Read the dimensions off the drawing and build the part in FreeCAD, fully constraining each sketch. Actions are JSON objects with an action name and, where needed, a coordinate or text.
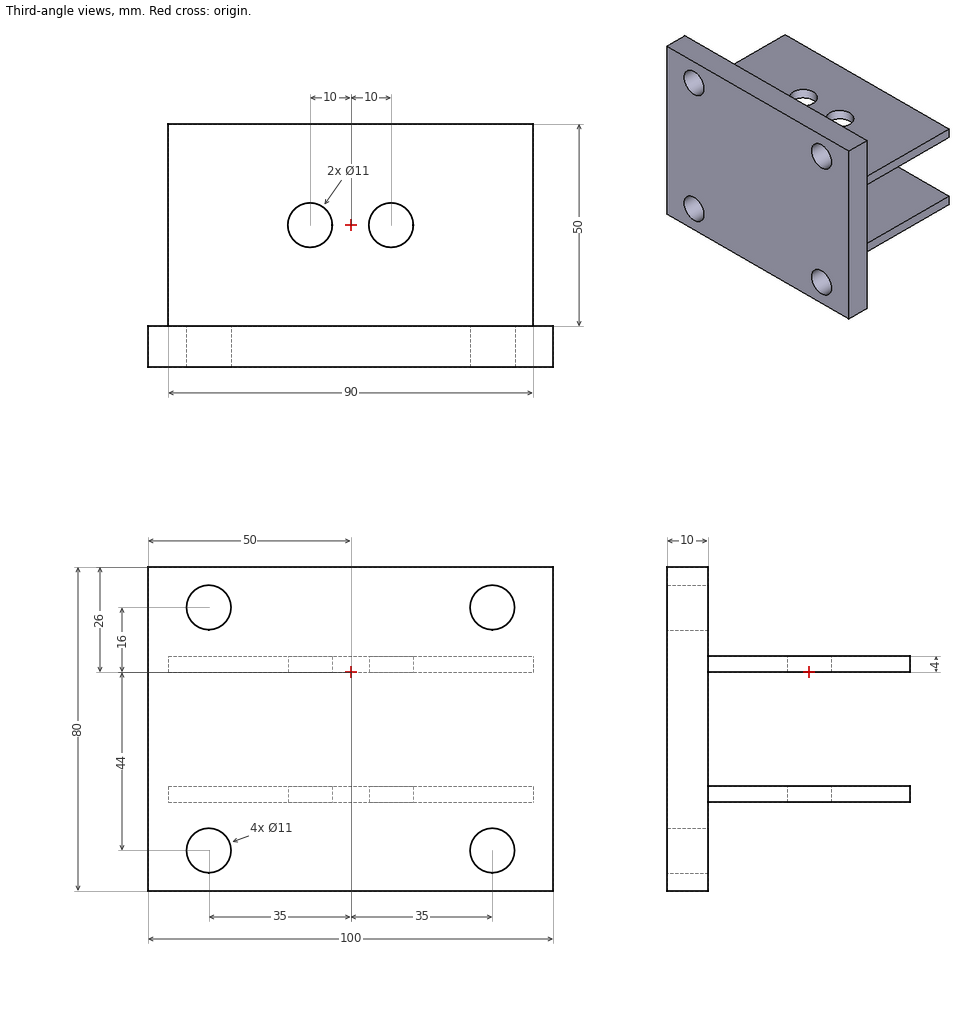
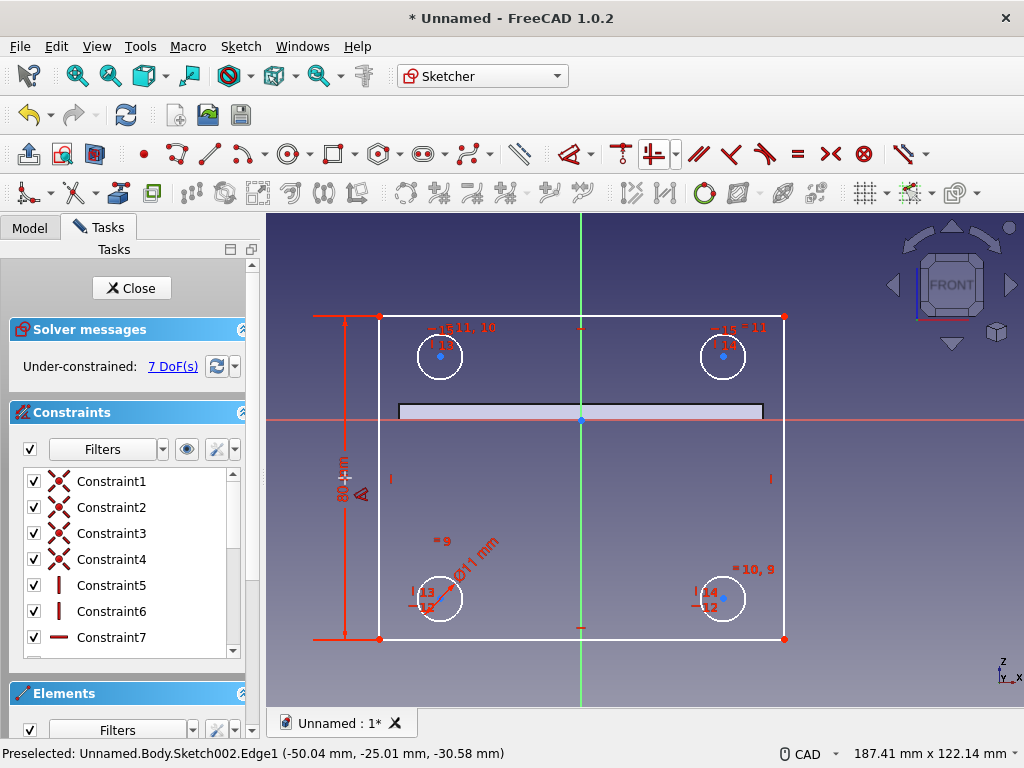
{"action": "left_click", "coordinate": [440, 599]}
{"action": "left_click", "coordinate": [511, 386]}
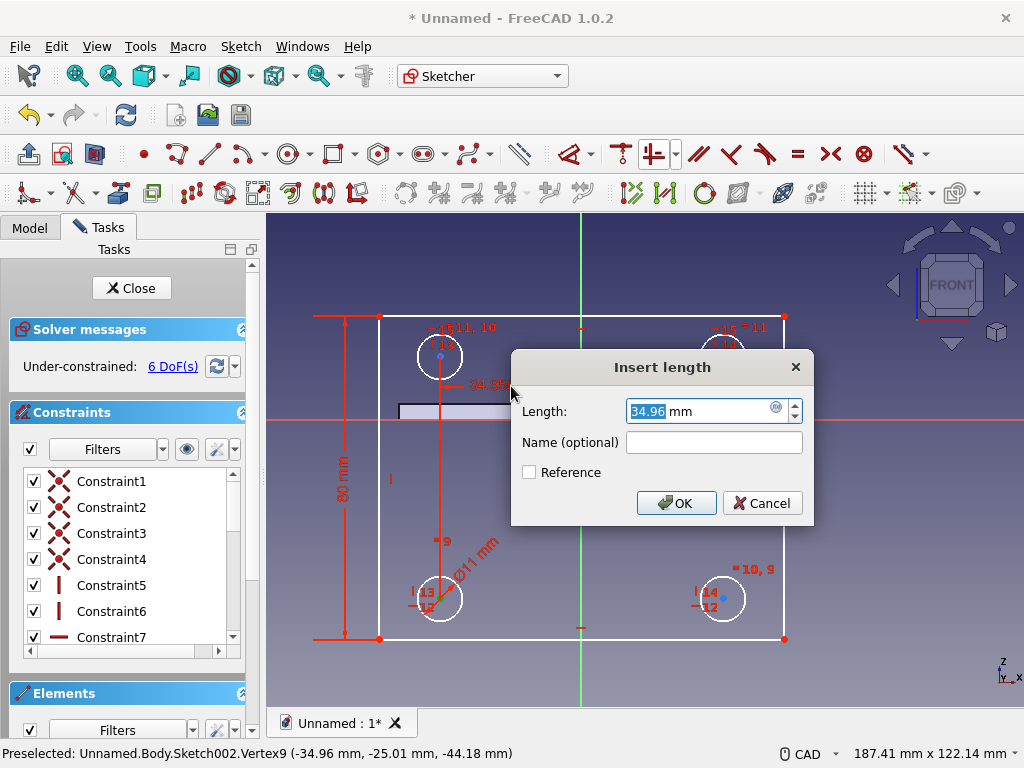
{"action": "type", "text": "35"}
{"action": "key", "text": "Return"}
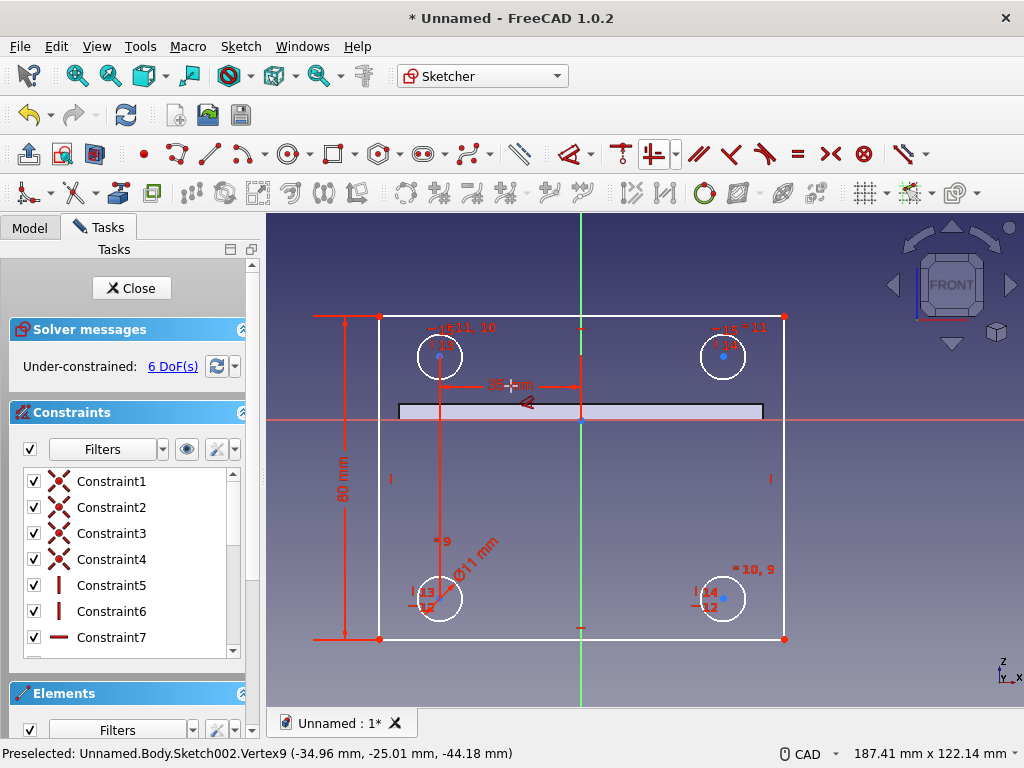
{"action": "left_click", "coordinate": [440, 599]}
{"action": "left_click", "coordinate": [406, 510]}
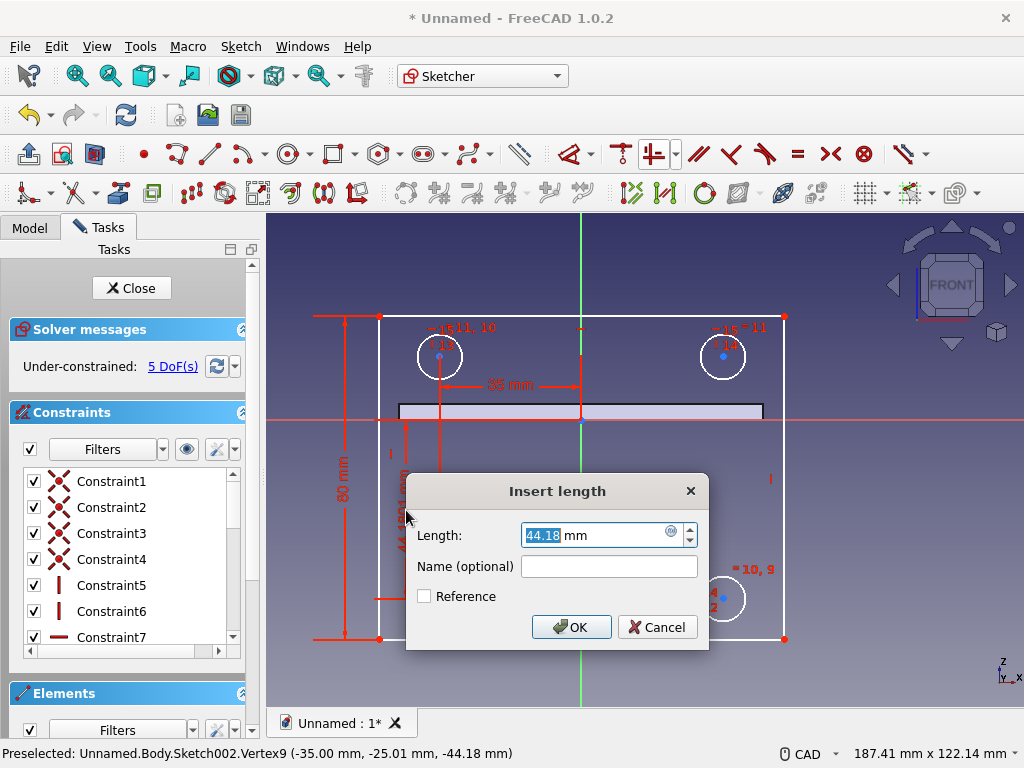
{"action": "type", "text": "44"}
{"action": "key", "text": "Return"}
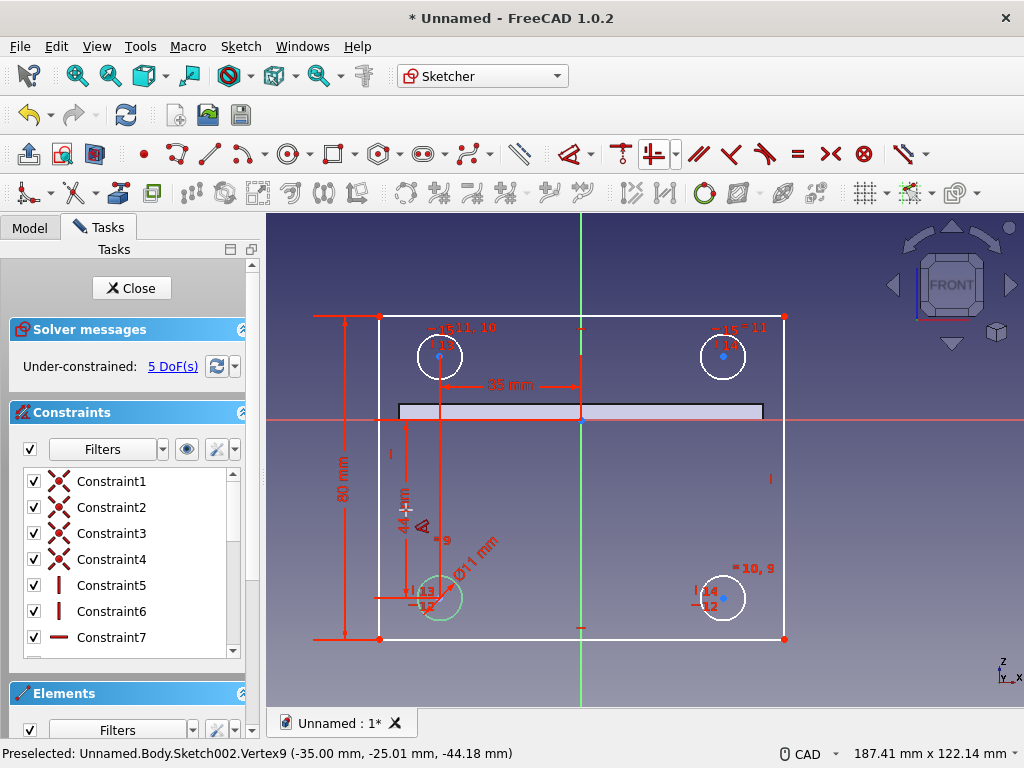
{"action": "left_click", "coordinate": [723, 598]}
{"action": "left_click", "coordinate": [652, 386]}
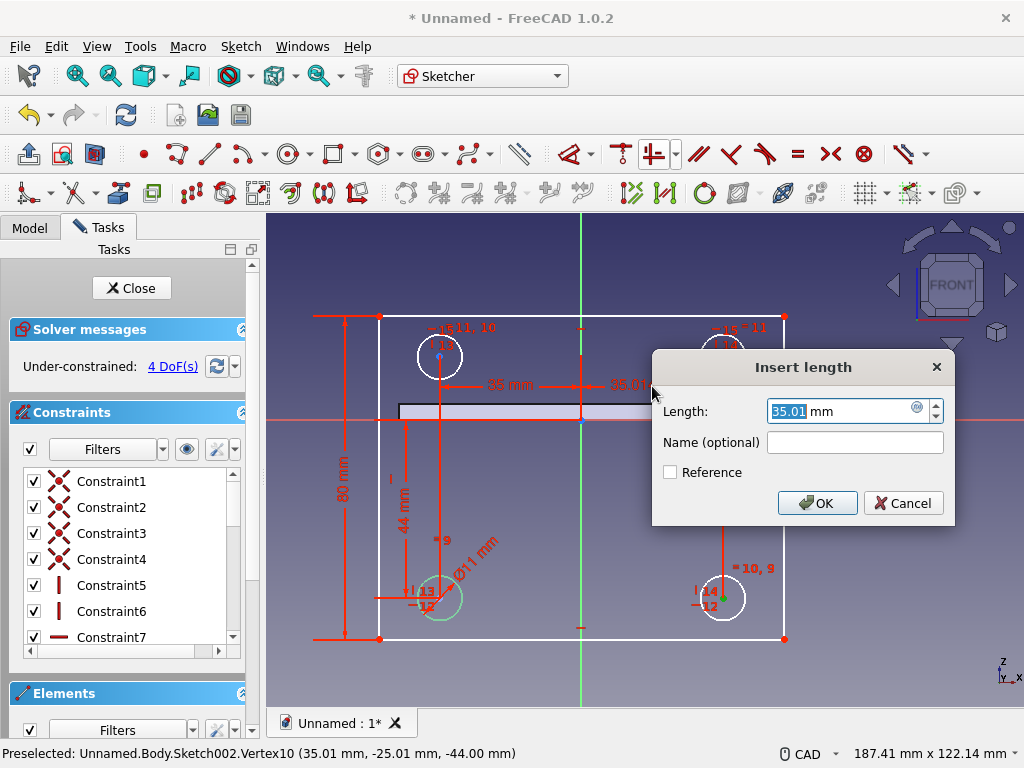
{"action": "type", "text": "35"}
{"action": "key", "text": "Return"}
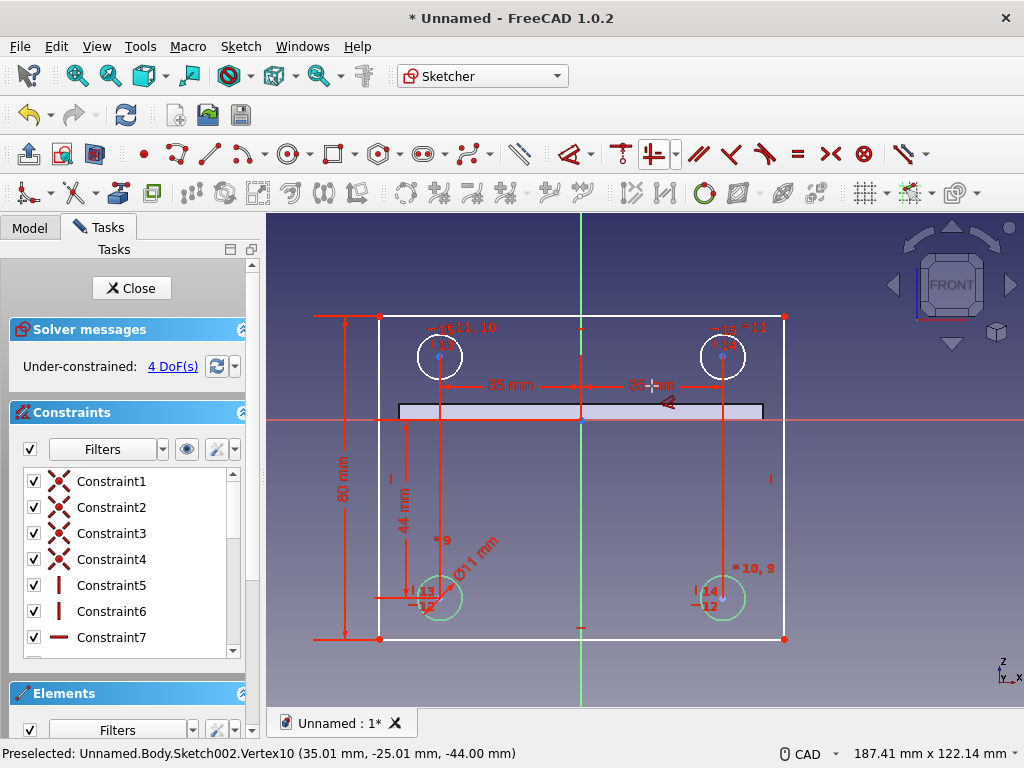
{"action": "left_click", "coordinate": [440, 357]}
{"action": "left_click", "coordinate": [406, 389]}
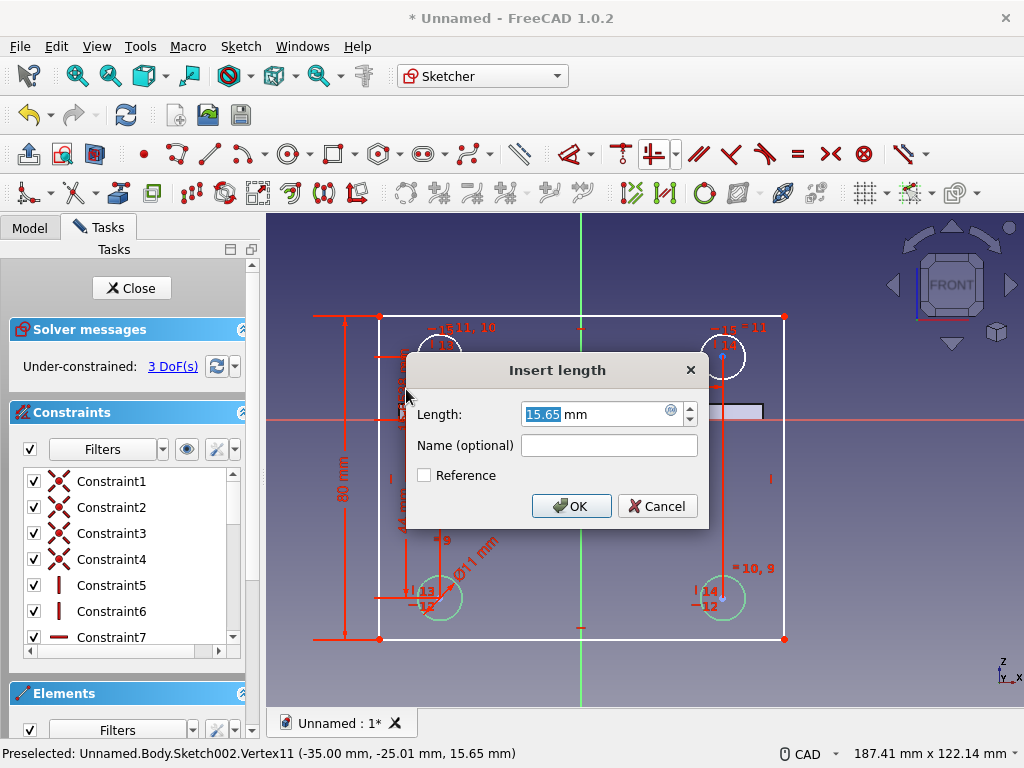
{"action": "type", "text": "16"}
{"action": "key", "text": "Return"}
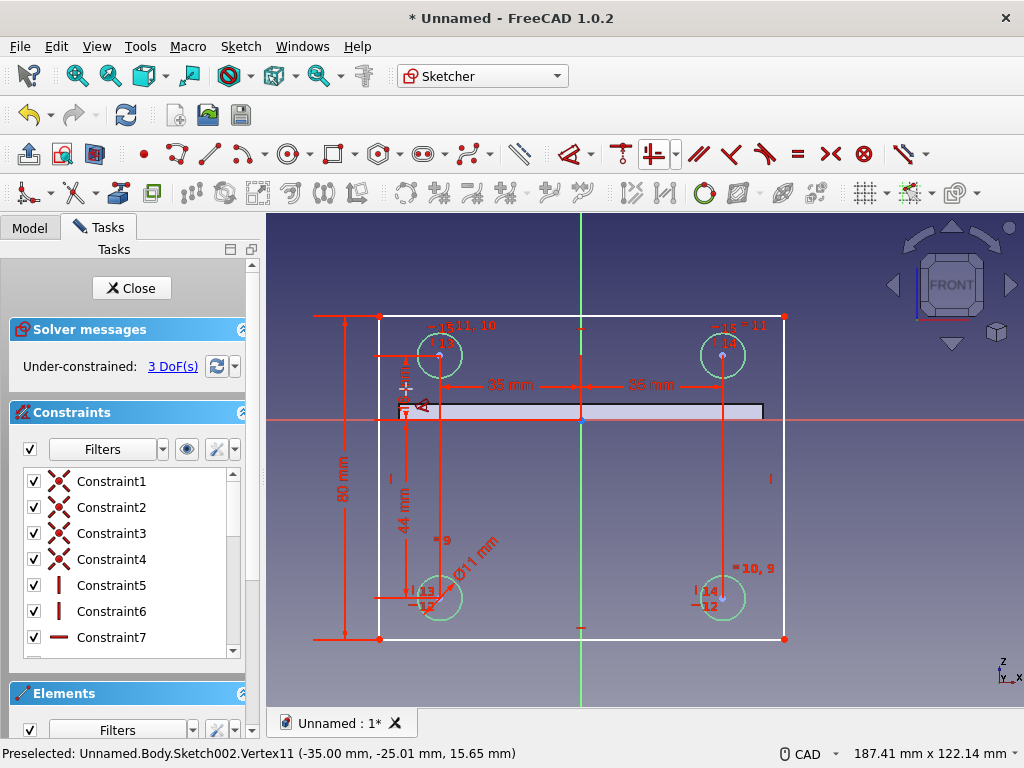
{"action": "left_click", "coordinate": [500, 640]}
{"action": "left_click", "coordinate": [488, 674]}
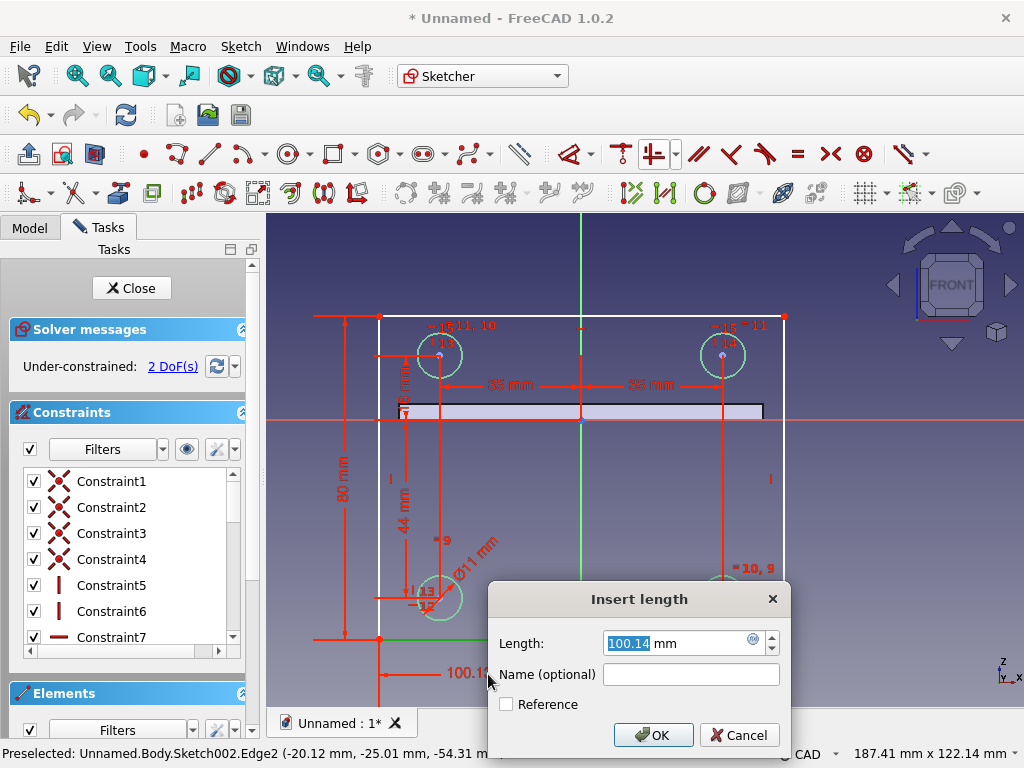
{"action": "type", "text": "100"}
{"action": "key", "text": "Return"}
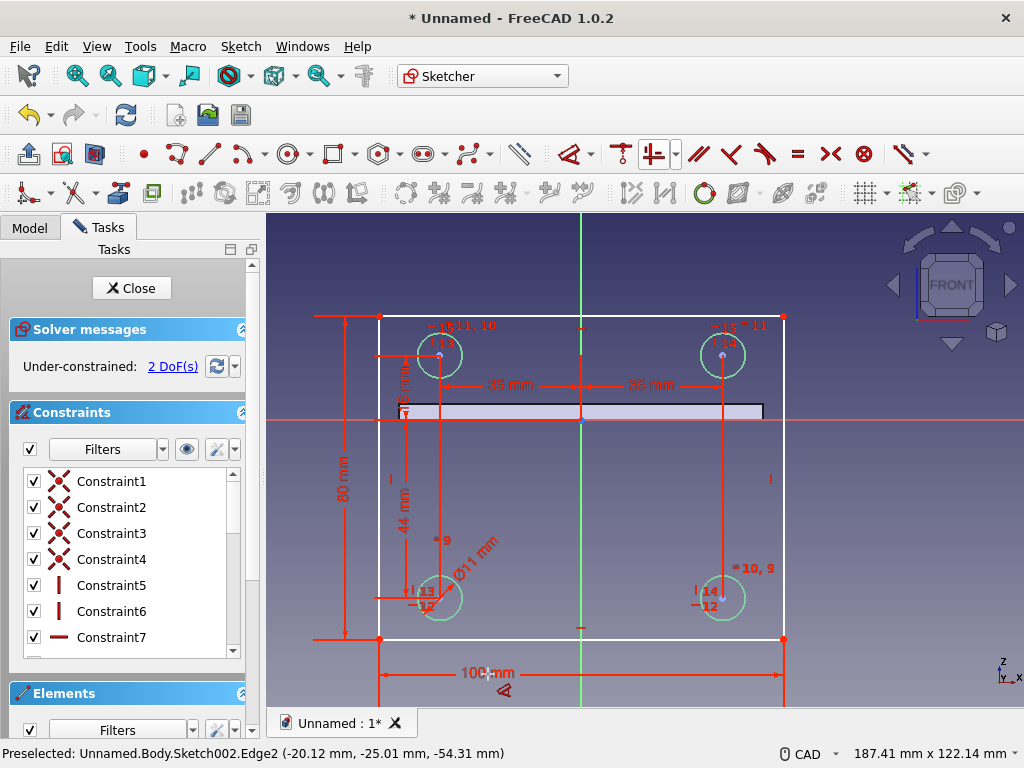
{"action": "left_click", "coordinate": [379, 316]}
{"action": "left_click", "coordinate": [480, 282]}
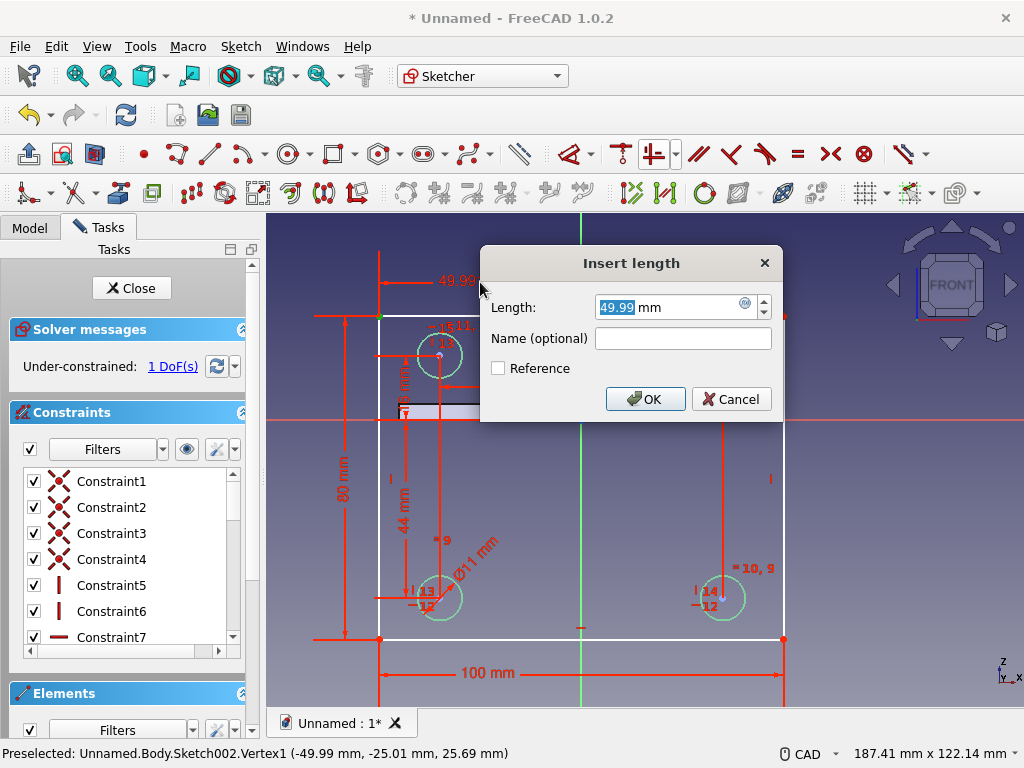
{"action": "type", "text": "50"}
{"action": "key", "text": "Return"}